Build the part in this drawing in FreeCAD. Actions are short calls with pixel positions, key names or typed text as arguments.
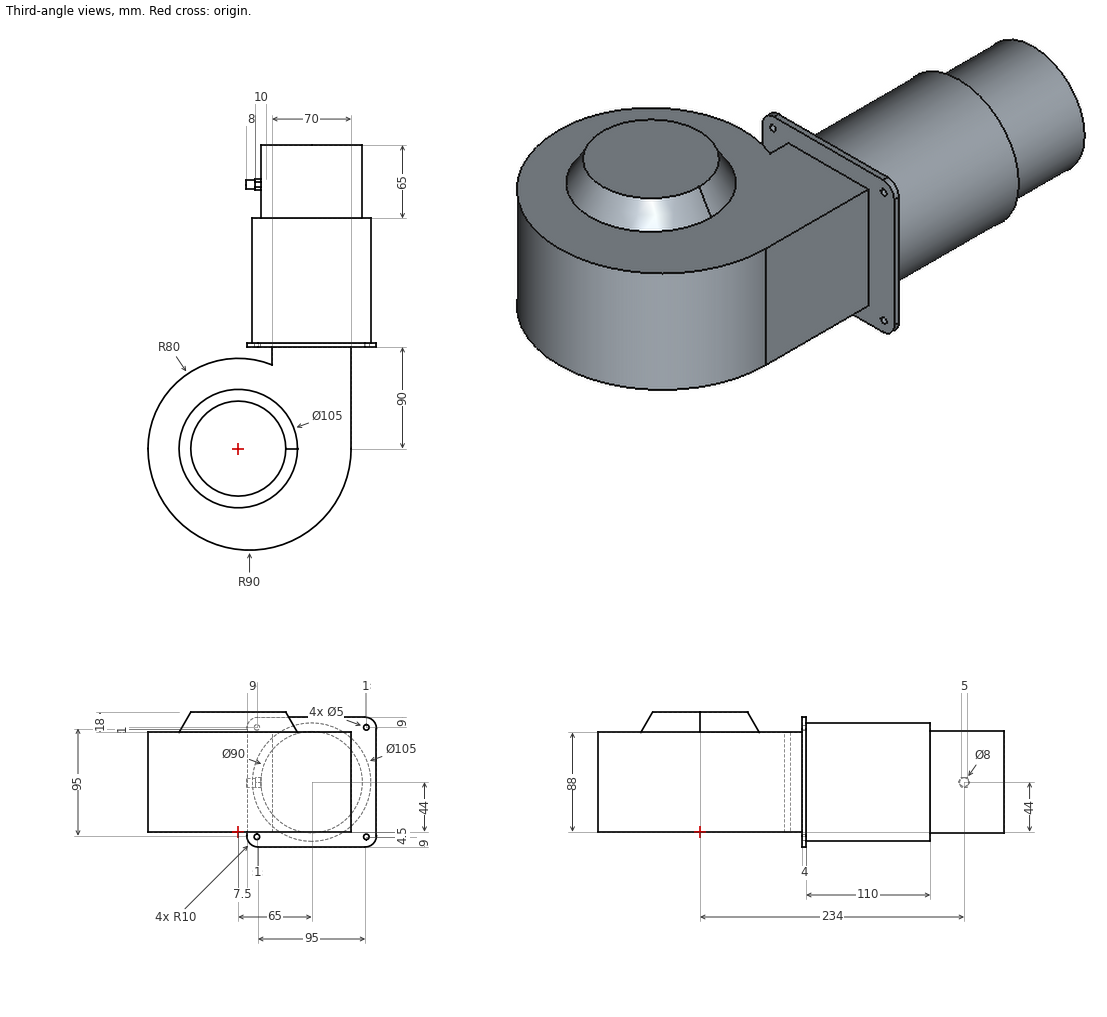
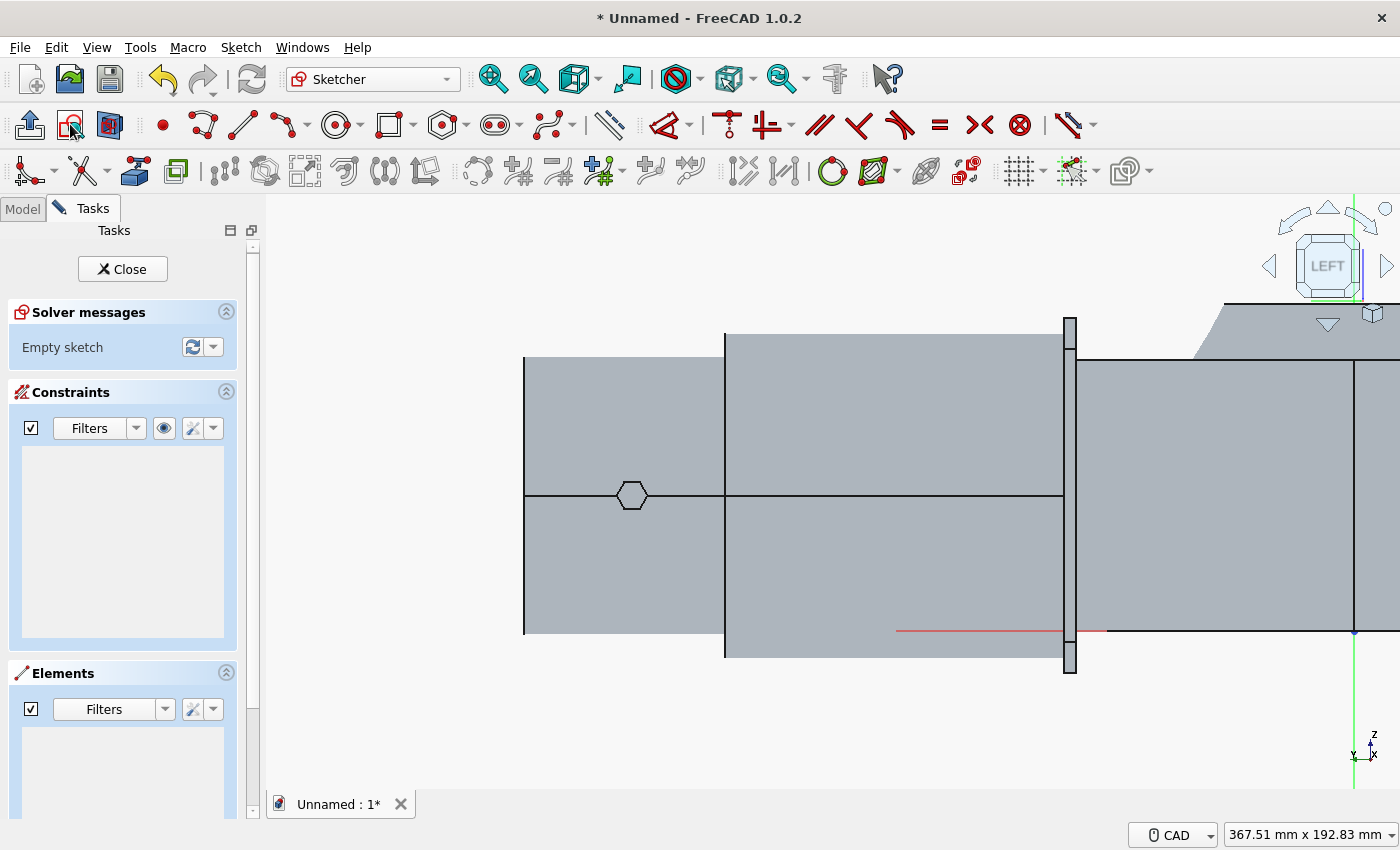
scroll(624, 496, up, 14)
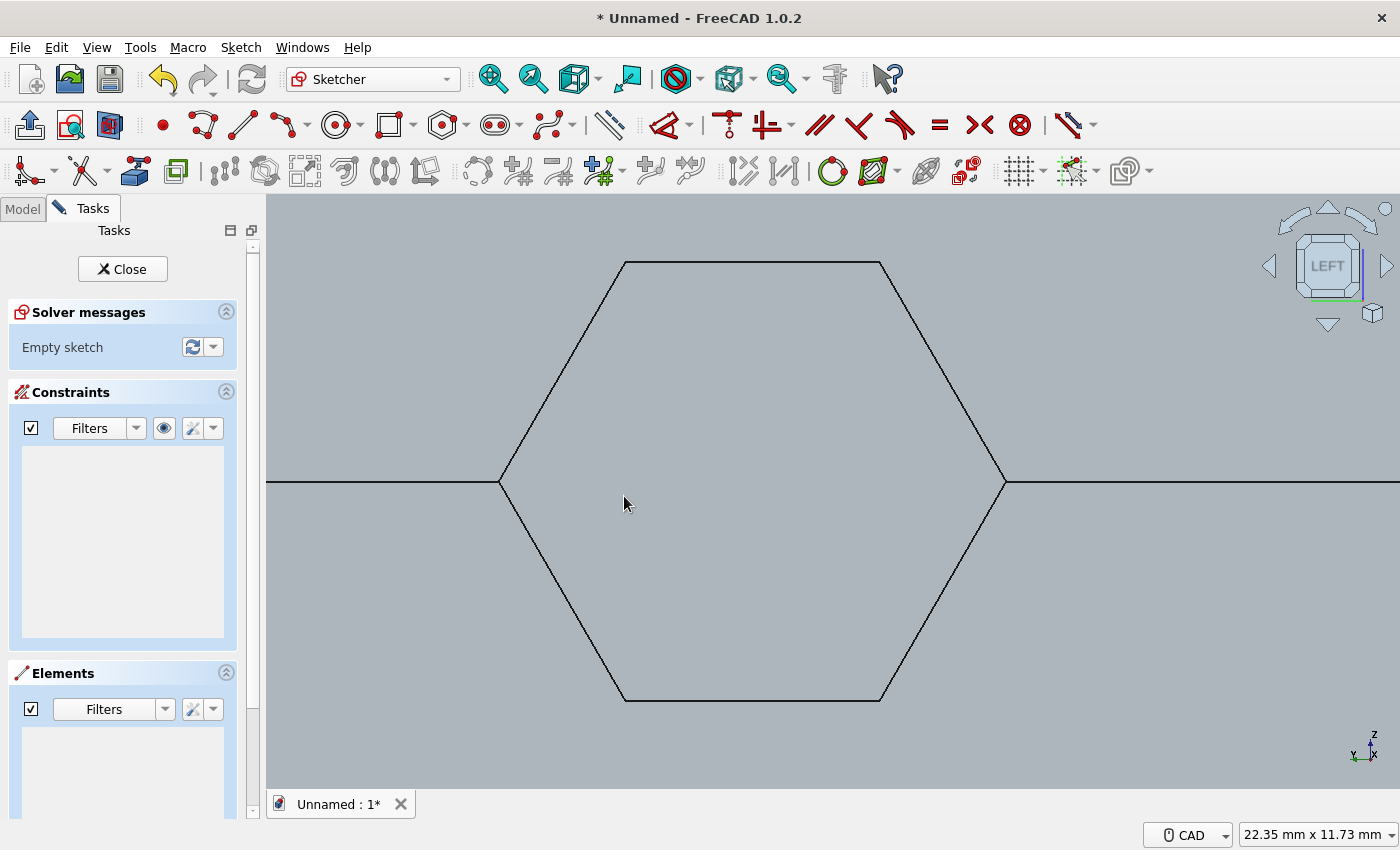
click(336, 126)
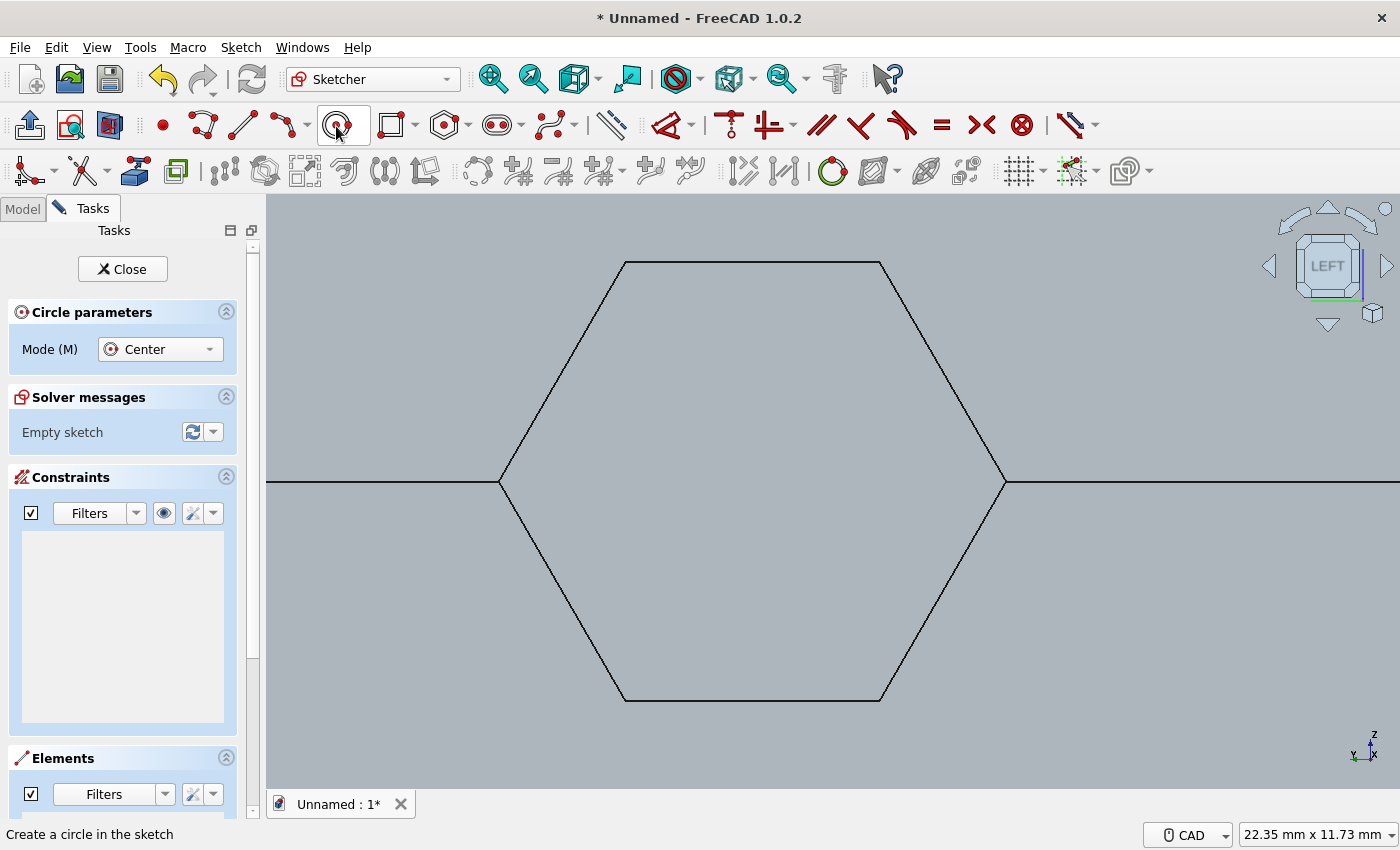
click(752, 482)
click(896, 338)
key(Escape)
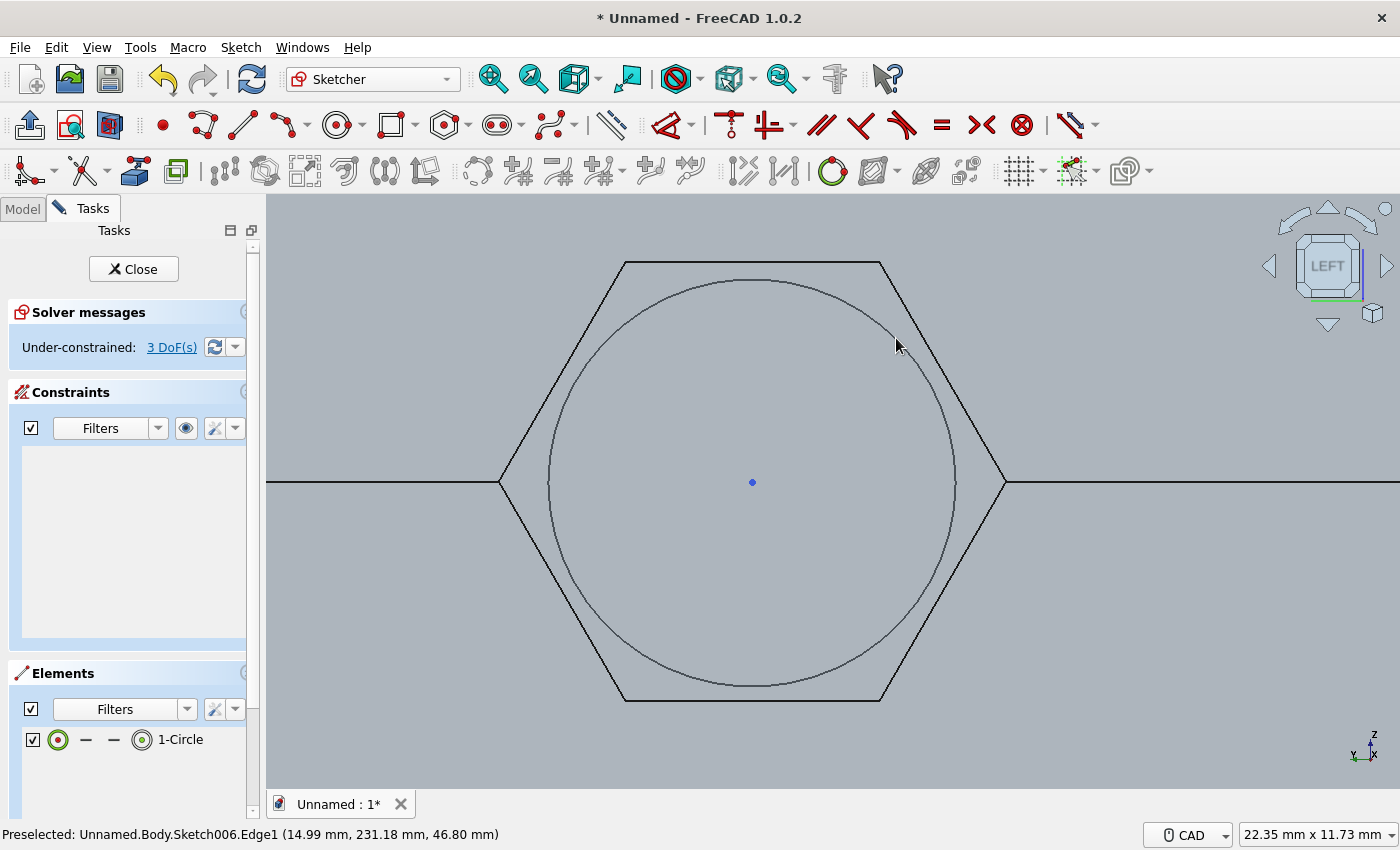
click(666, 126)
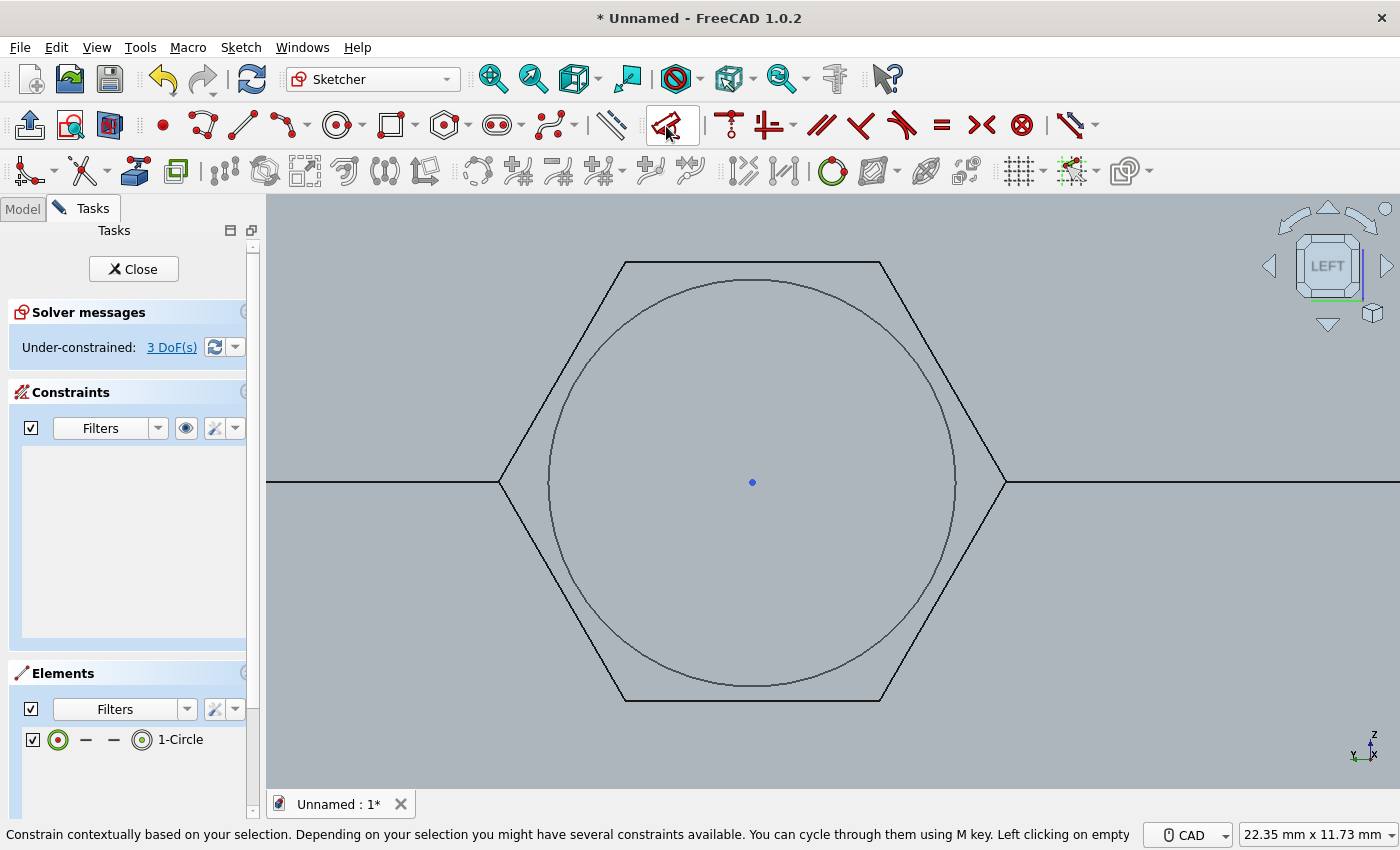
click(896, 339)
click(919, 316)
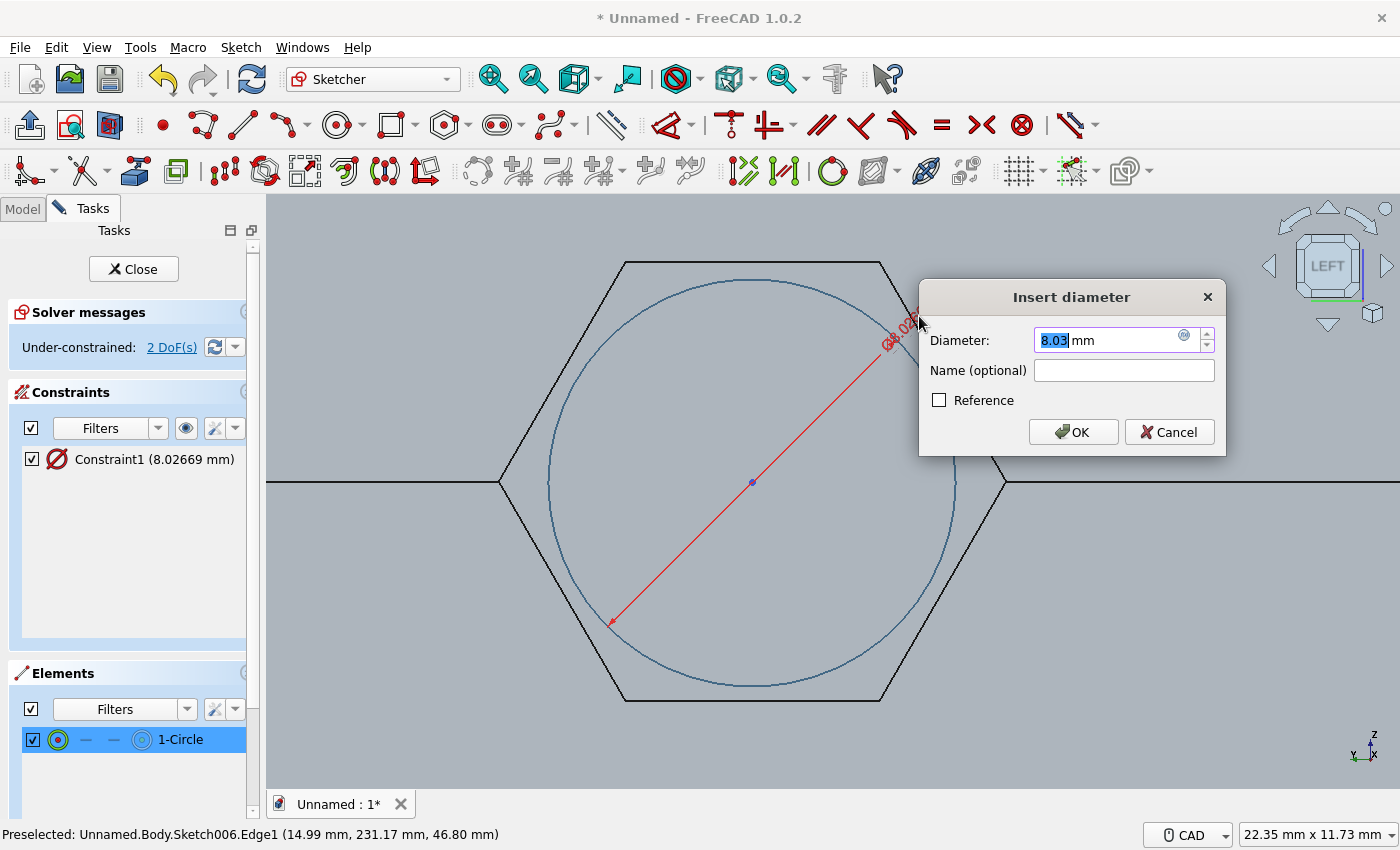
text(8)
key(Return)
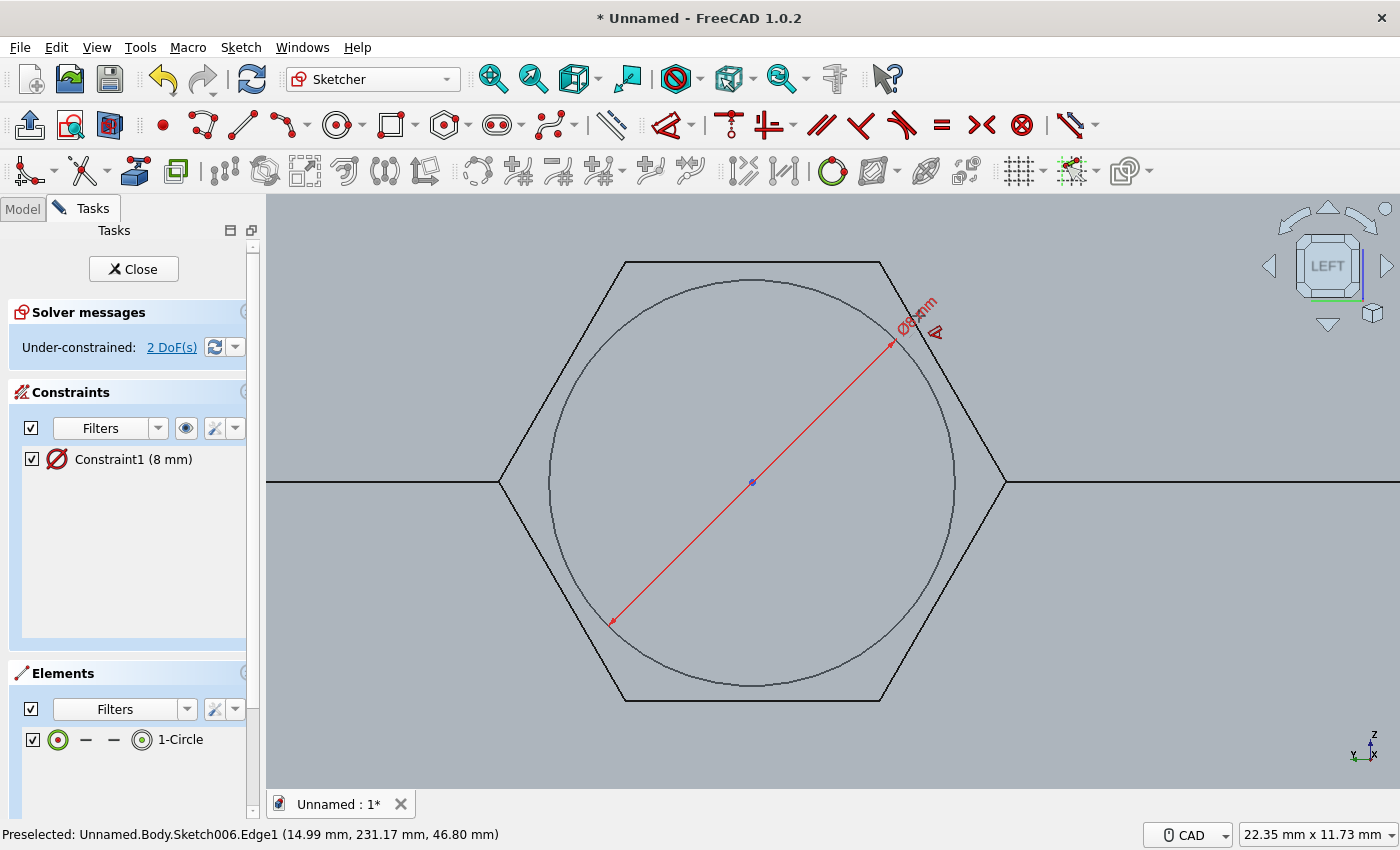
click(752, 483)
click(718, 622)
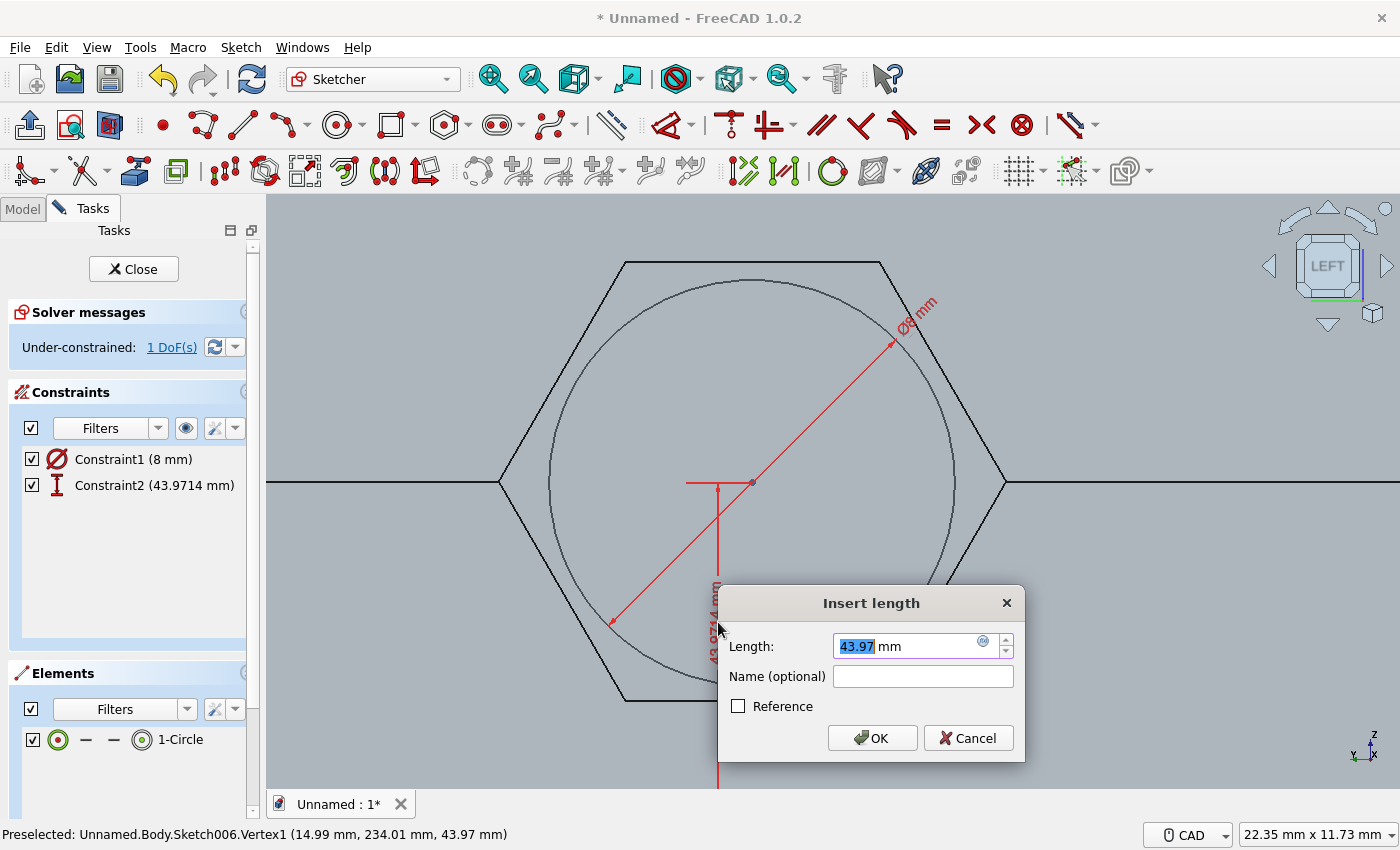
text(44)
key(Return)